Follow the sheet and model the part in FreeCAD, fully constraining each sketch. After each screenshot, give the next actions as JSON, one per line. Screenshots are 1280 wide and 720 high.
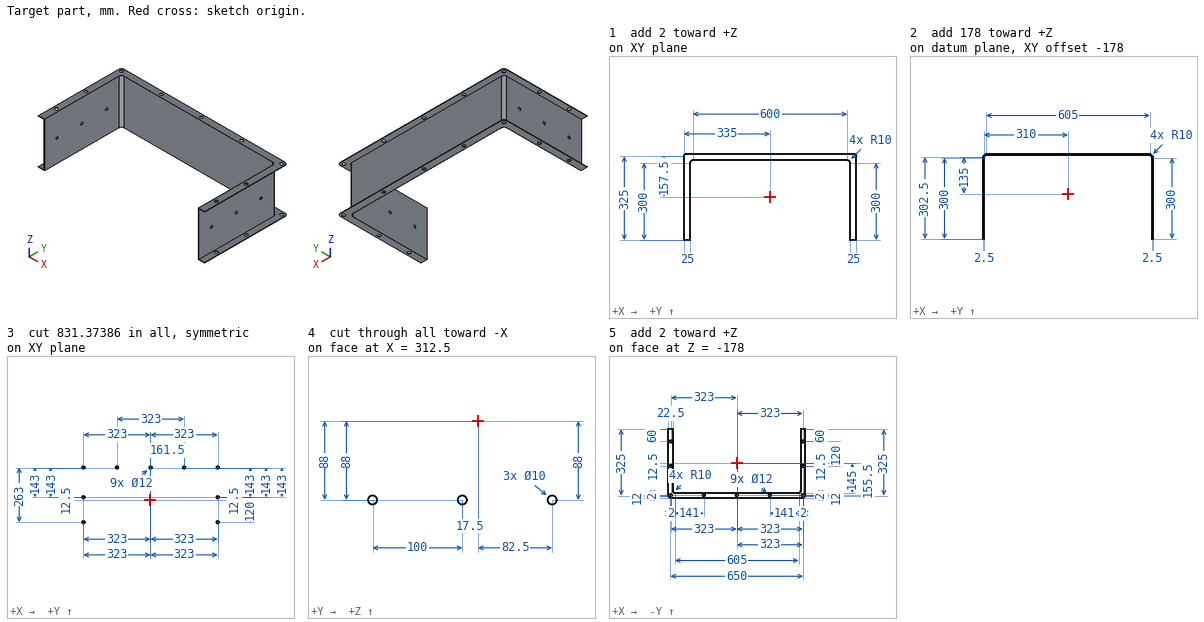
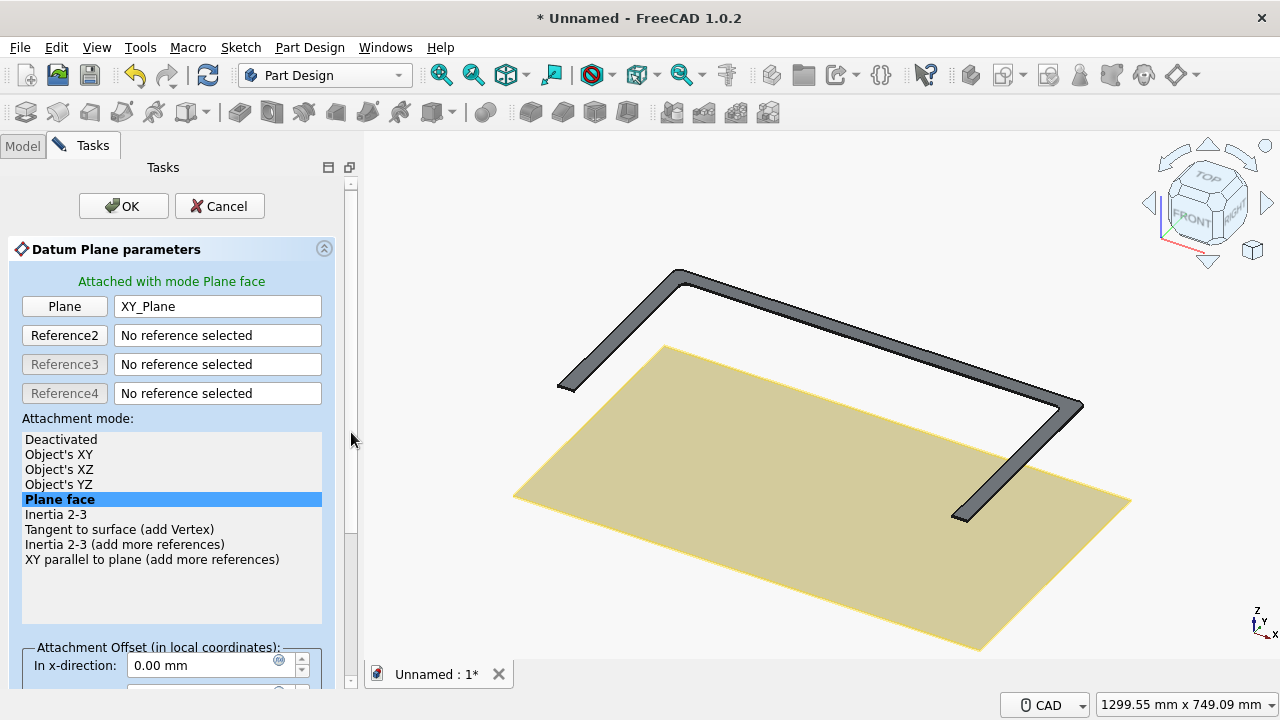
{"action": "left_click", "coordinate": [124, 206]}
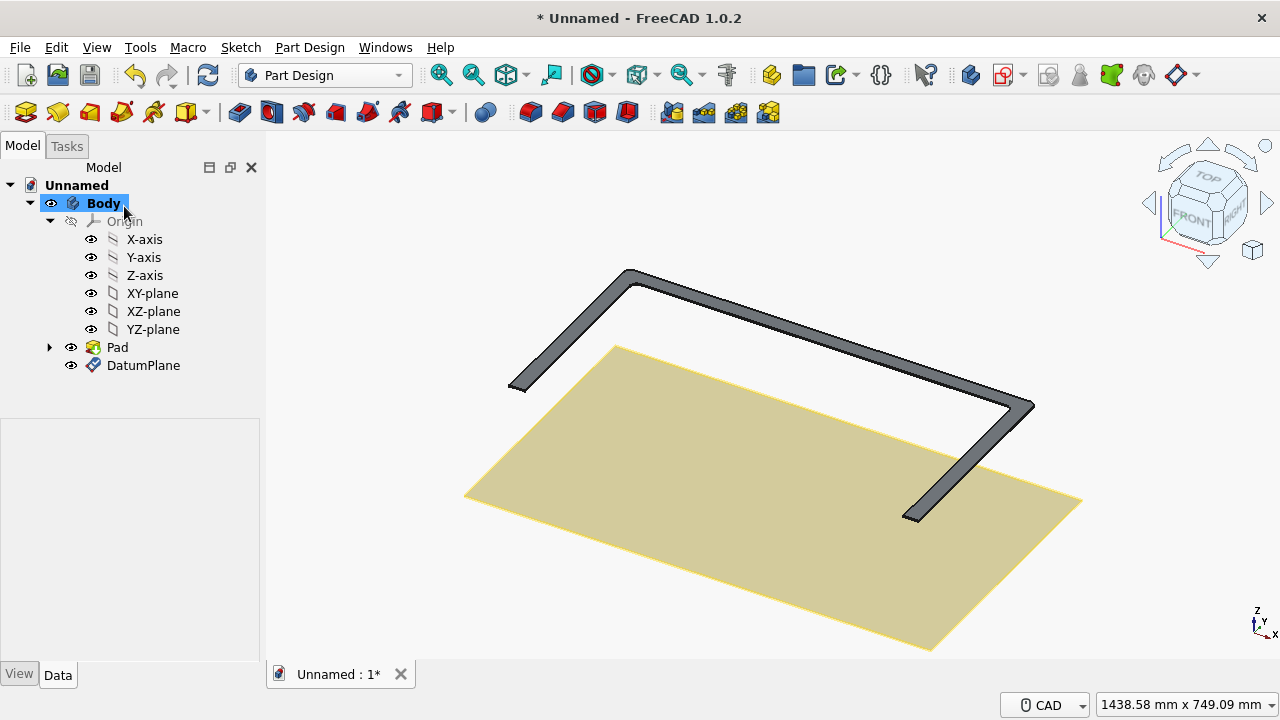
{"action": "left_click", "coordinate": [116, 365]}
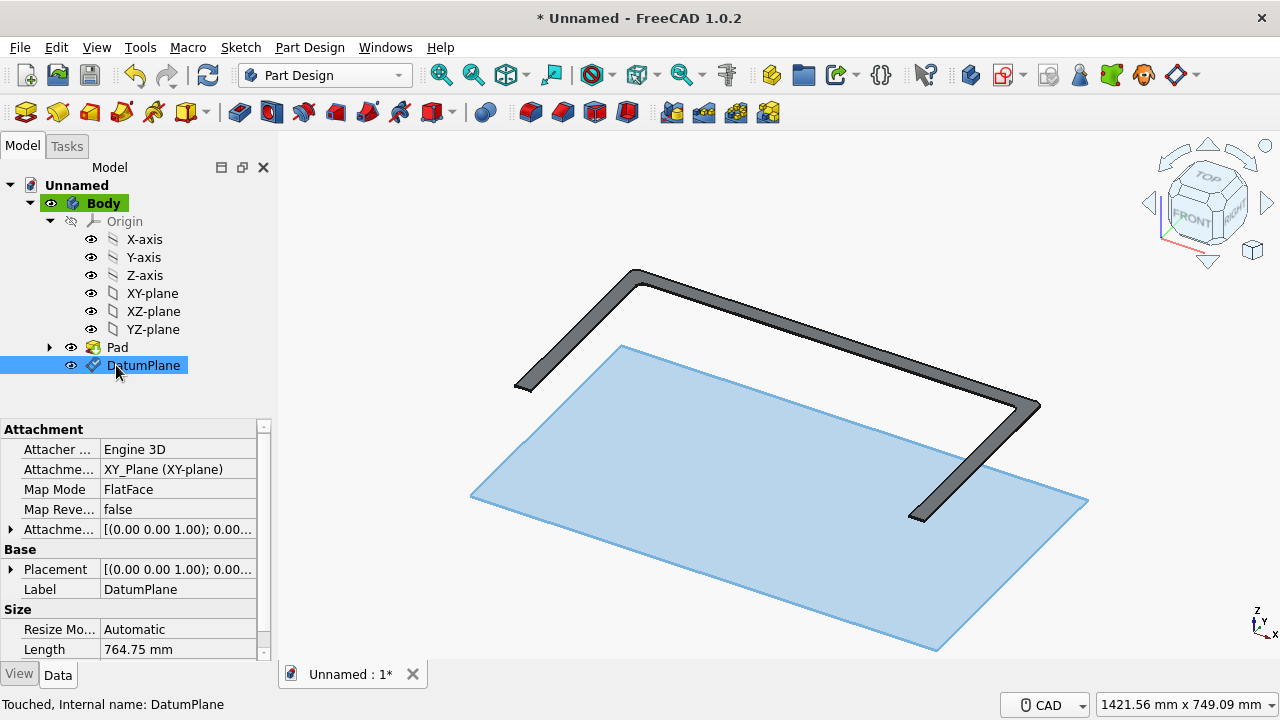
{"action": "left_click", "coordinate": [1004, 76]}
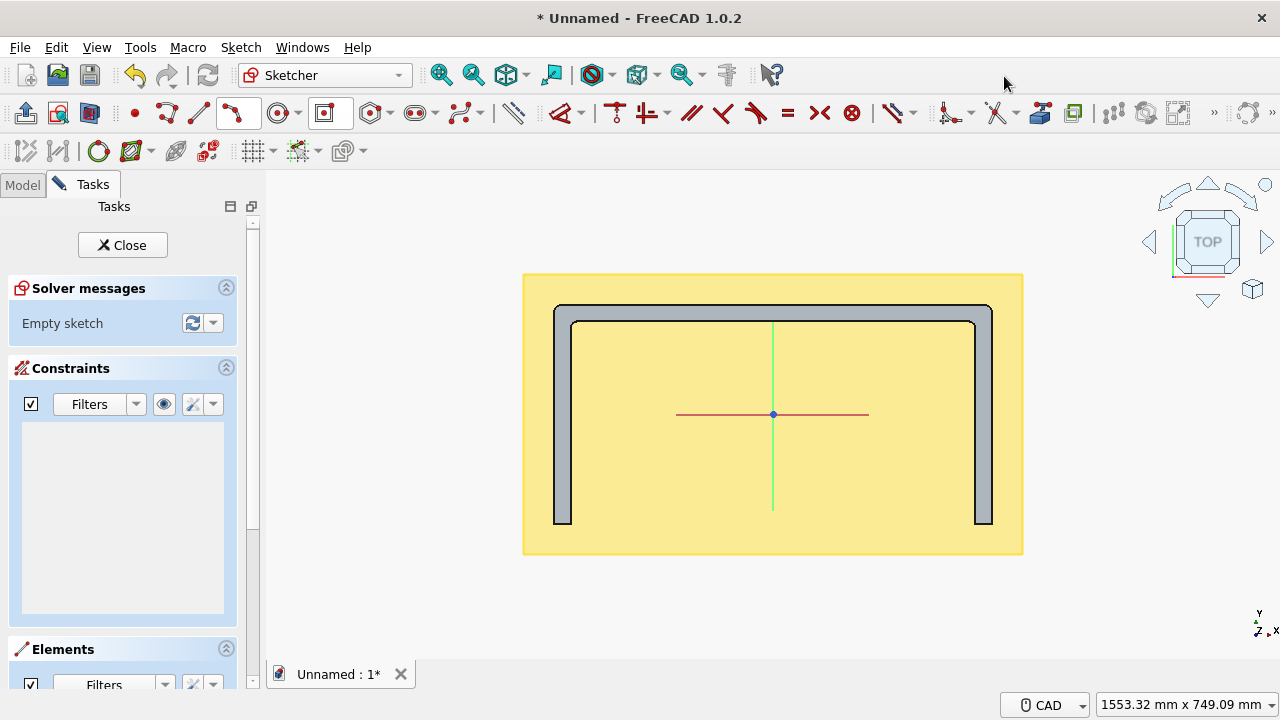
{"action": "left_click", "coordinate": [90, 114]}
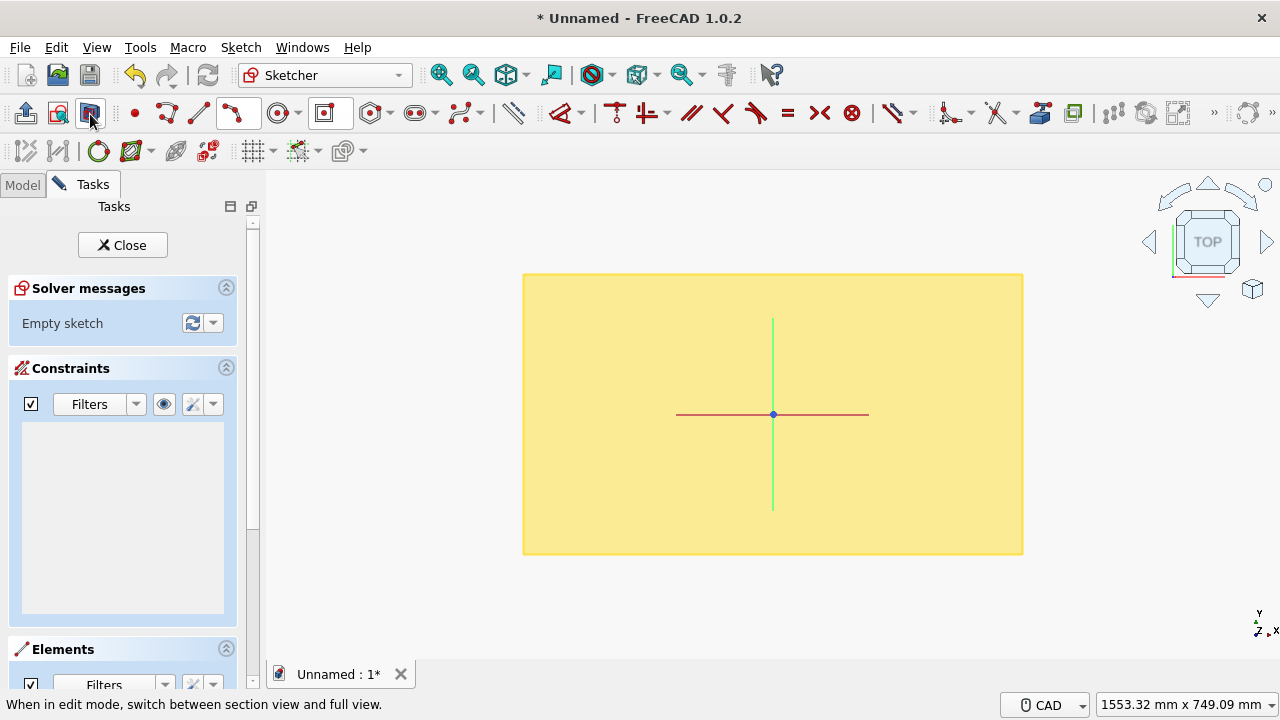
{"action": "scroll", "coordinate": [912, 437], "scroll_direction": "up", "scroll_amount": 2}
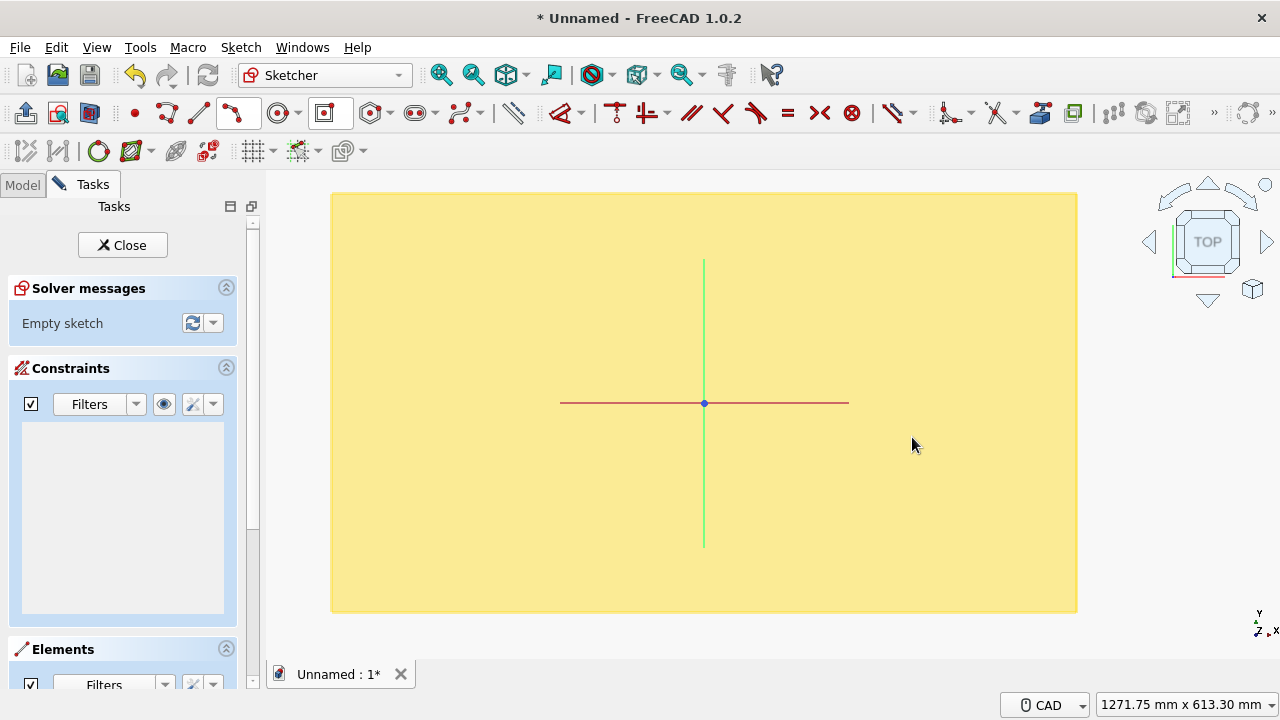
{"action": "left_click", "coordinate": [168, 114]}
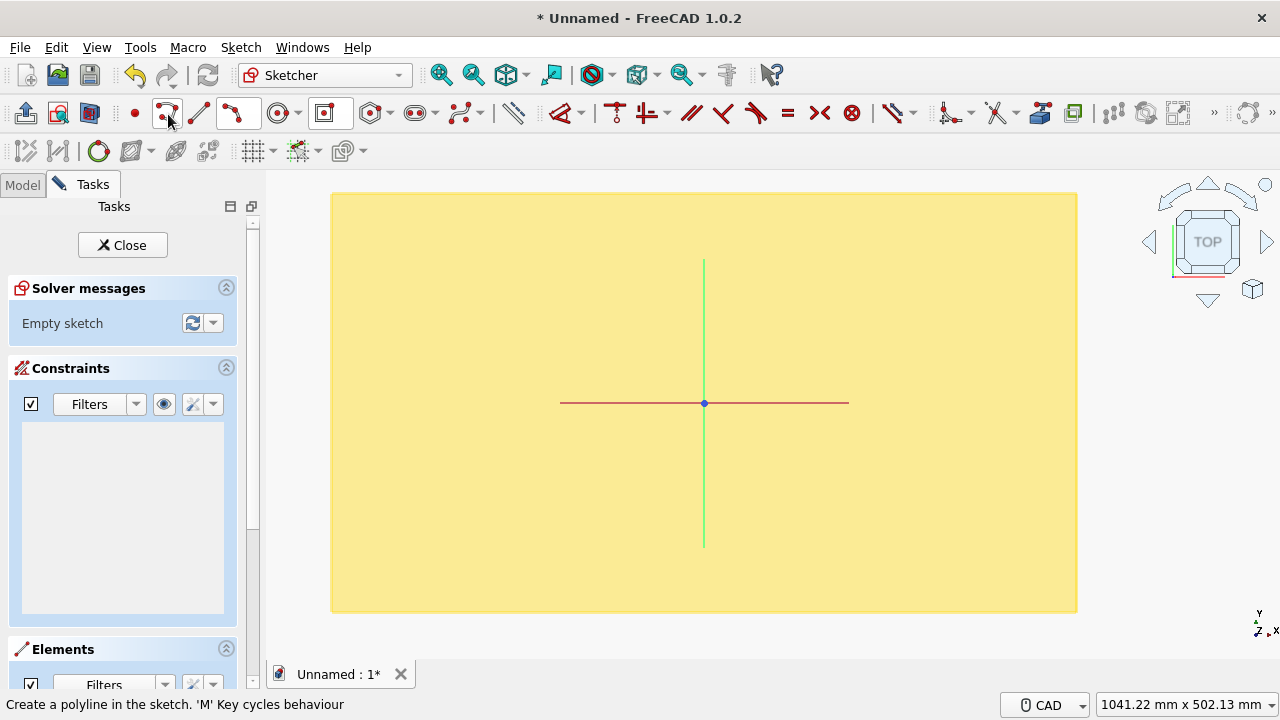
{"action": "left_click", "coordinate": [402, 274]}
{"action": "left_click", "coordinate": [402, 566]}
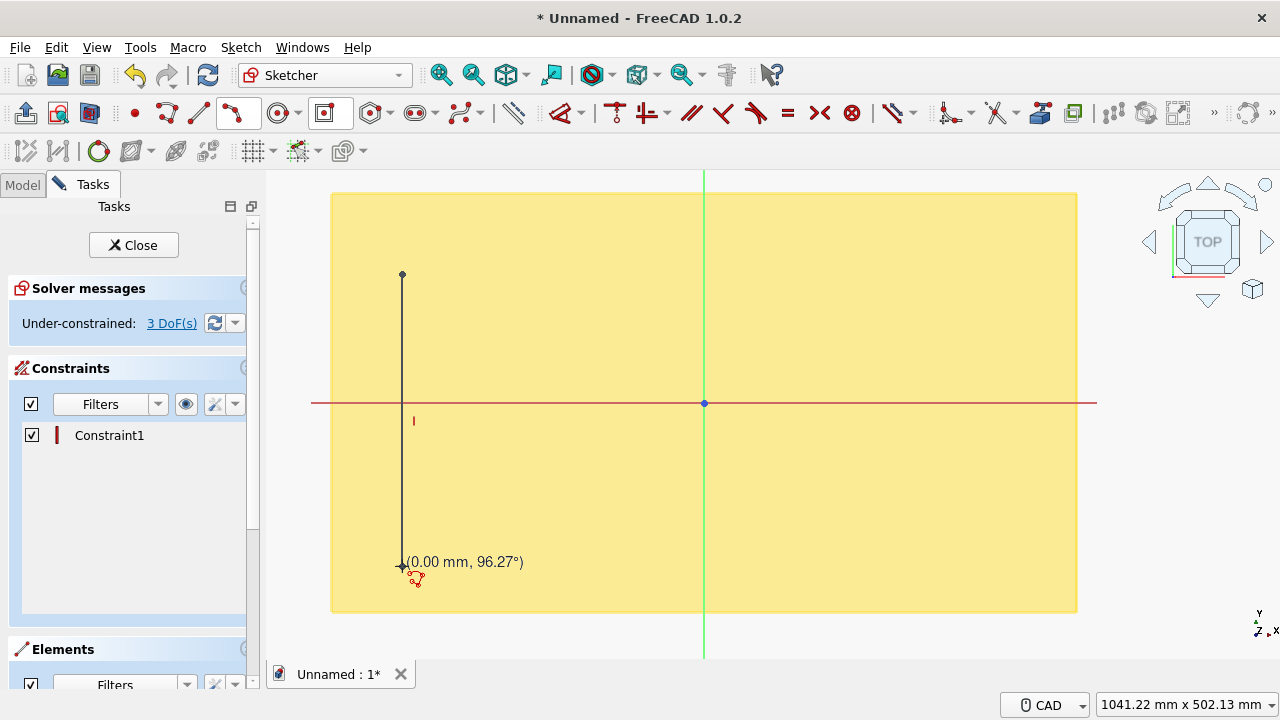
{"action": "scroll", "coordinate": [400, 566], "scroll_direction": "up", "scroll_amount": 10}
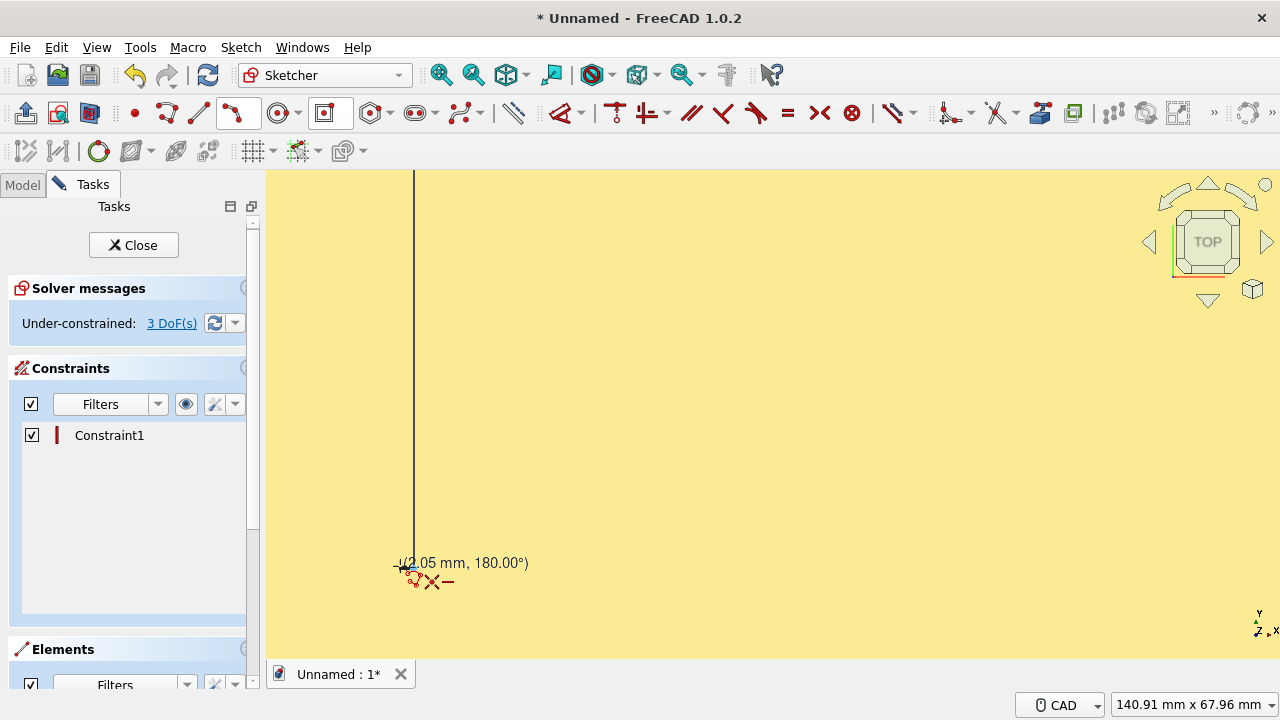
{"action": "left_click", "coordinate": [399, 561]}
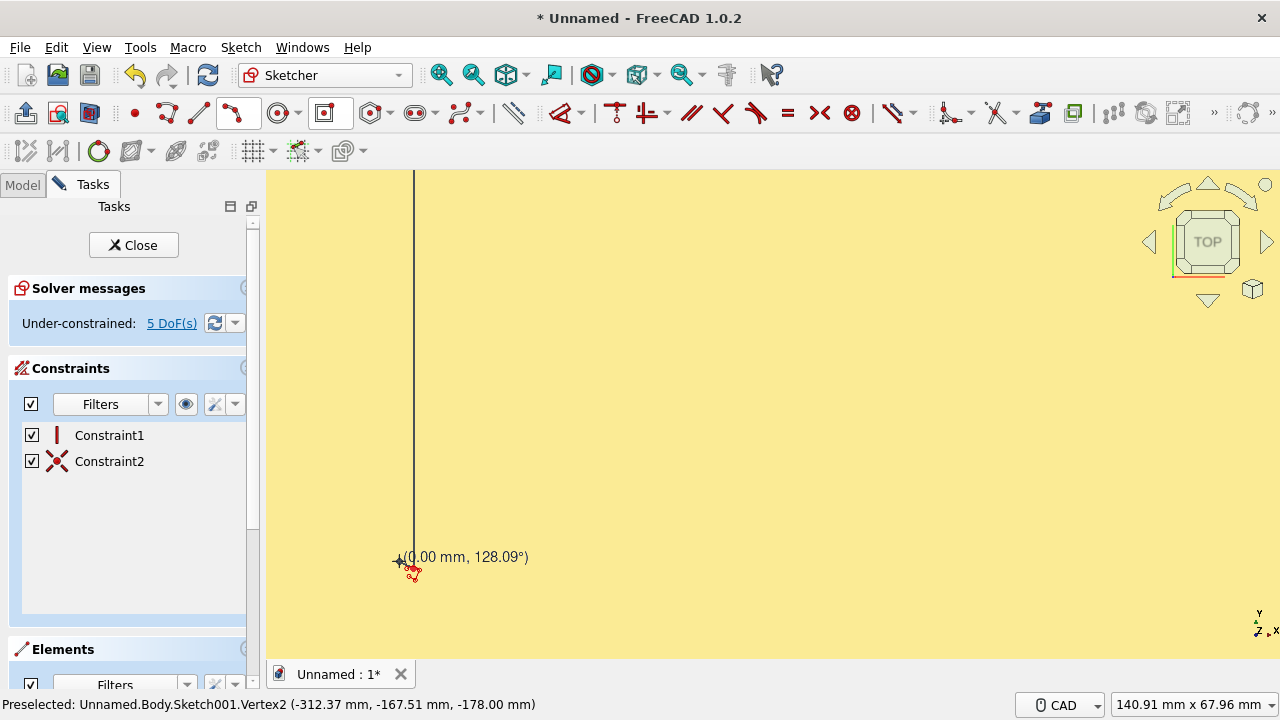
{"action": "scroll", "coordinate": [400, 567], "scroll_direction": "down", "scroll_amount": 10}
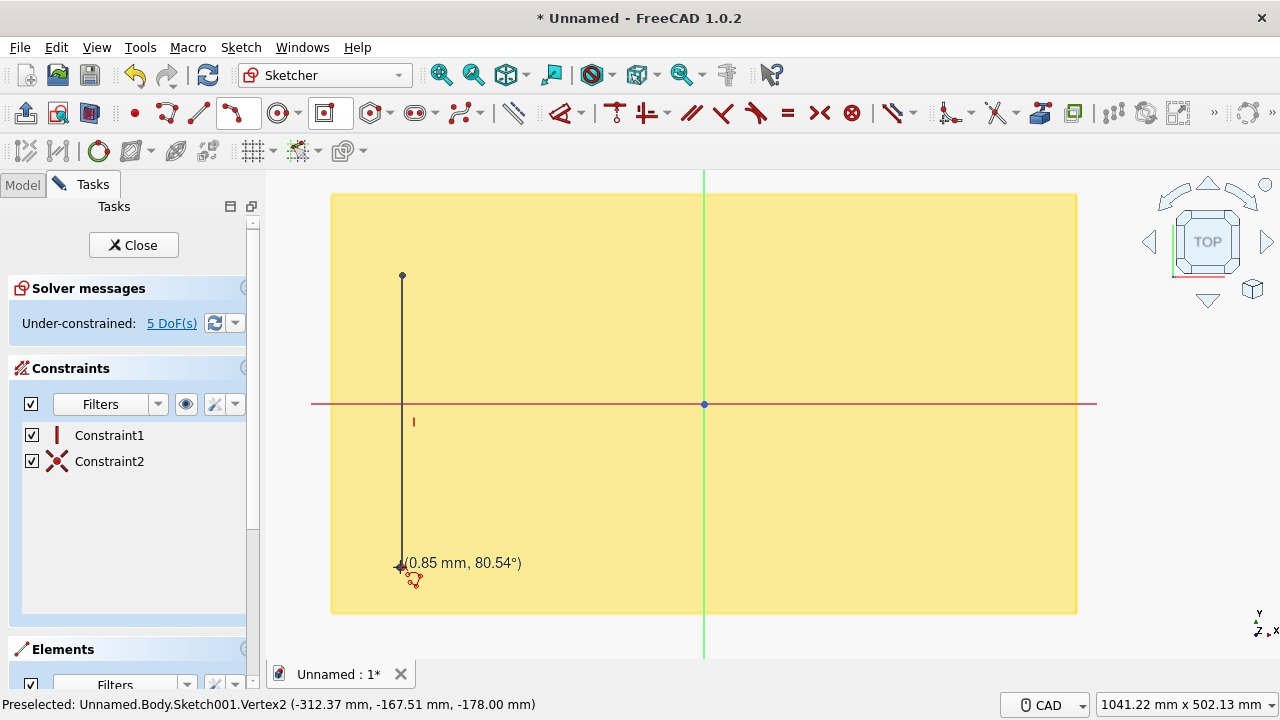
{"action": "scroll", "coordinate": [400, 273], "scroll_direction": "up", "scroll_amount": 8}